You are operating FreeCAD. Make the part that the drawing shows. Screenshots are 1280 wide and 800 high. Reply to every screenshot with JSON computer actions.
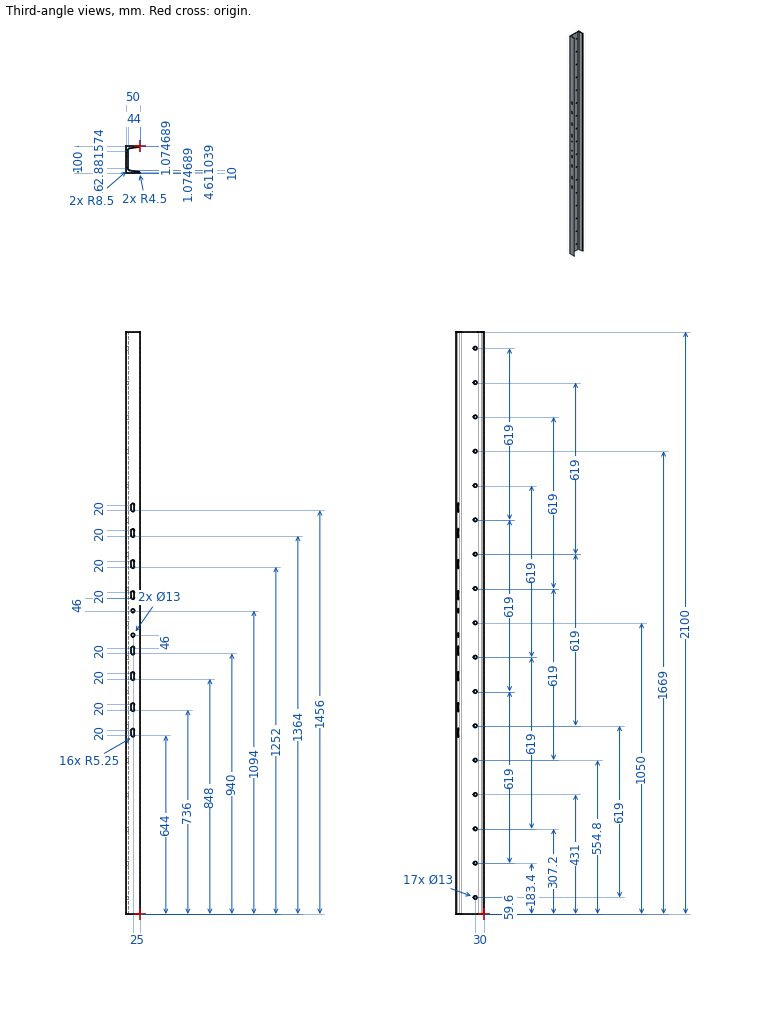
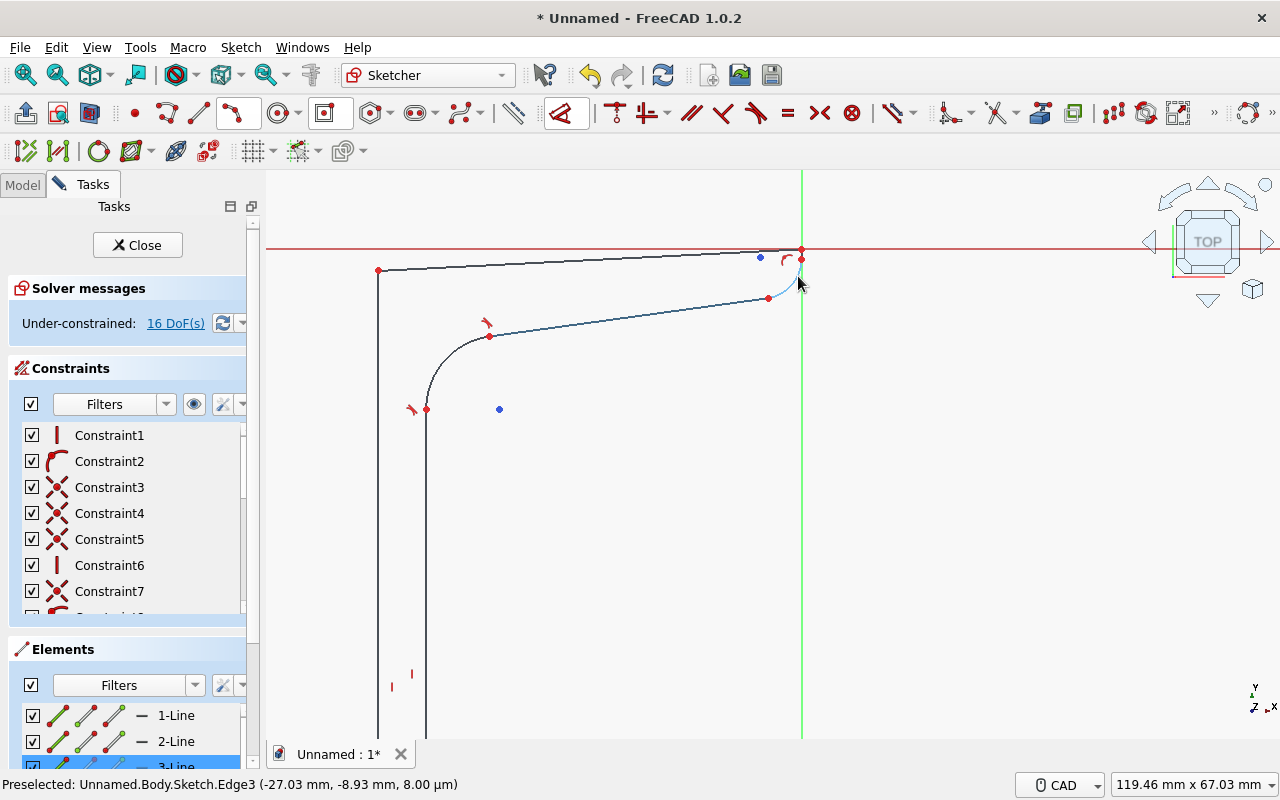
{"action": "left_click", "coordinate": [798, 275]}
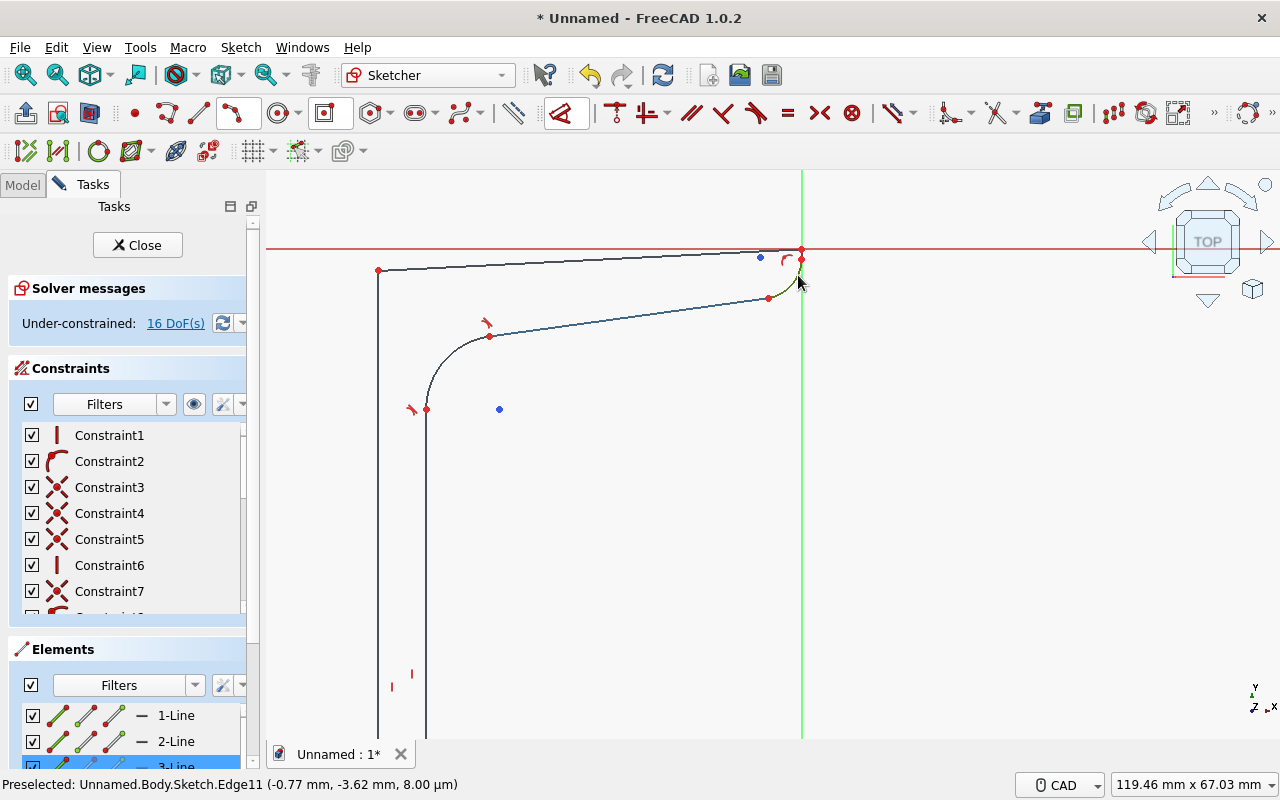
{"action": "left_click", "coordinate": [756, 114]}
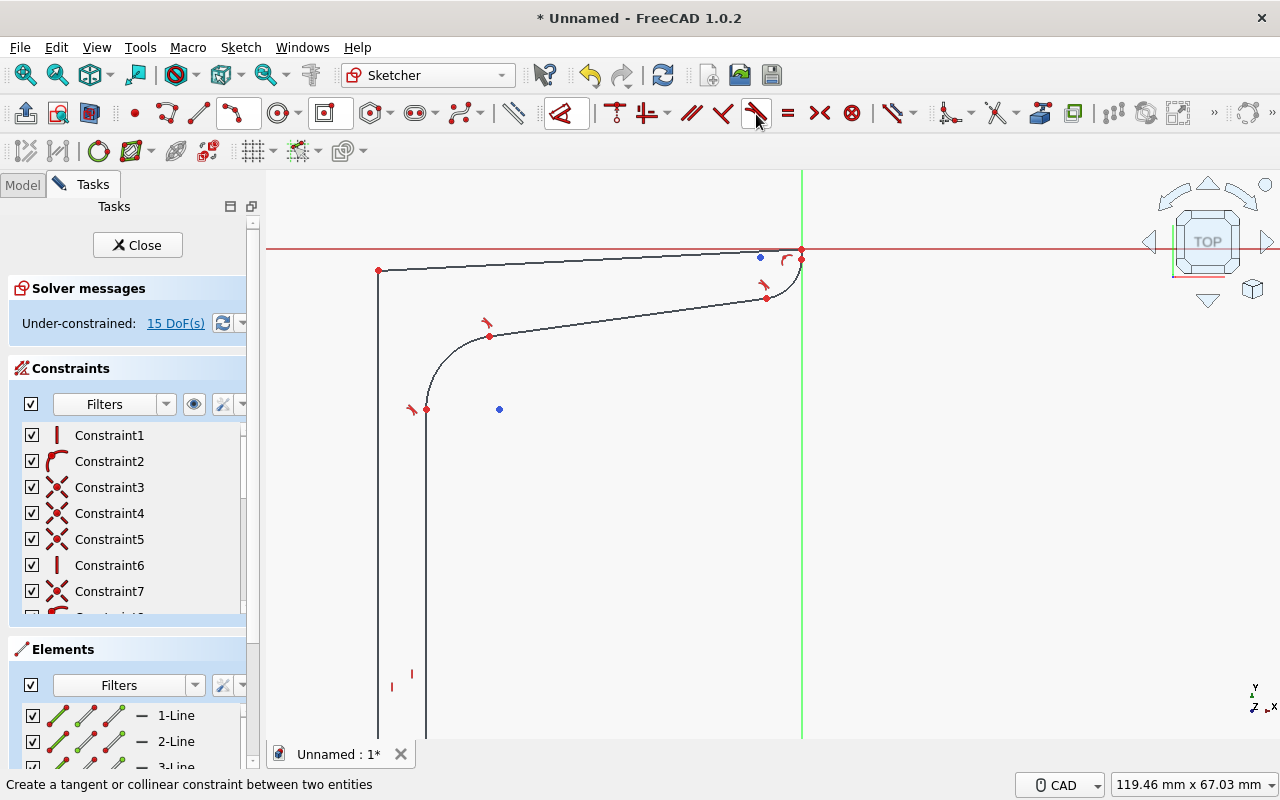
{"action": "scroll", "coordinate": [802, 254], "scroll_direction": "up", "scroll_amount": 6}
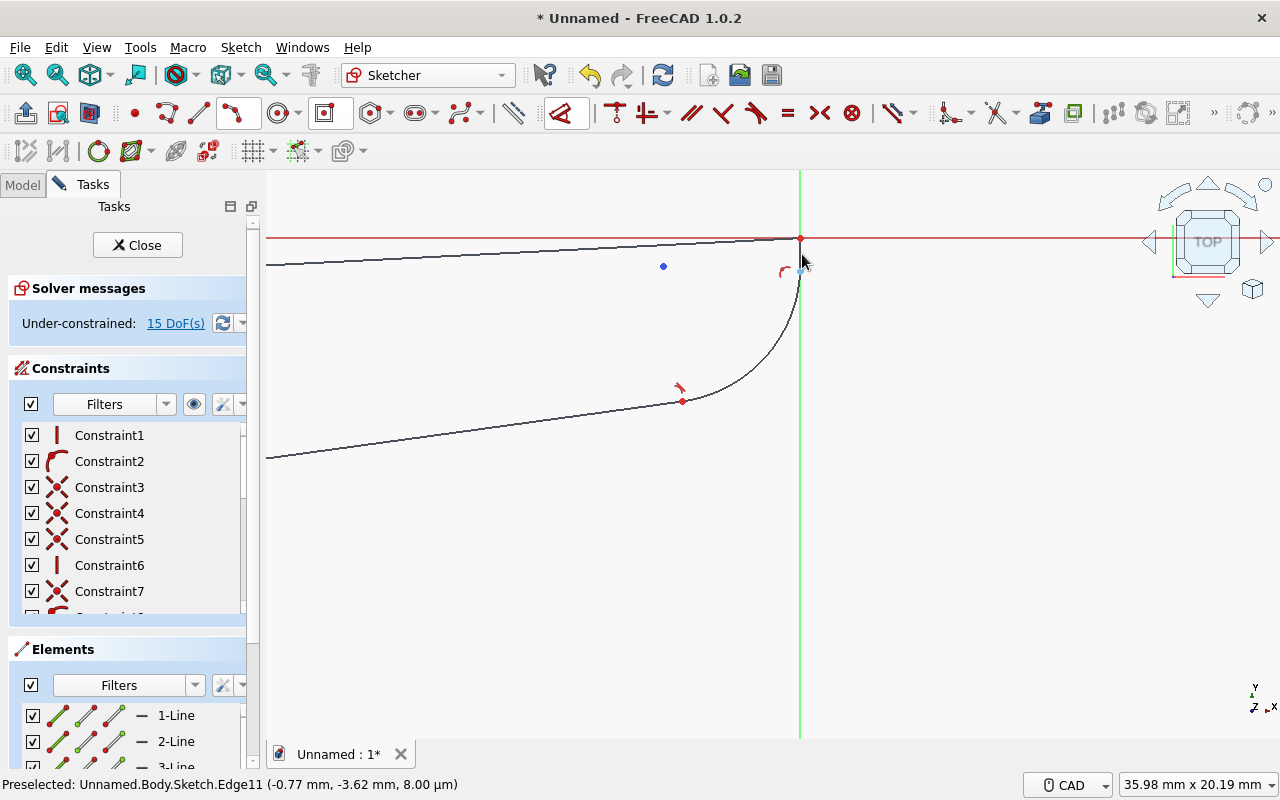
{"action": "left_click", "coordinate": [800, 255]}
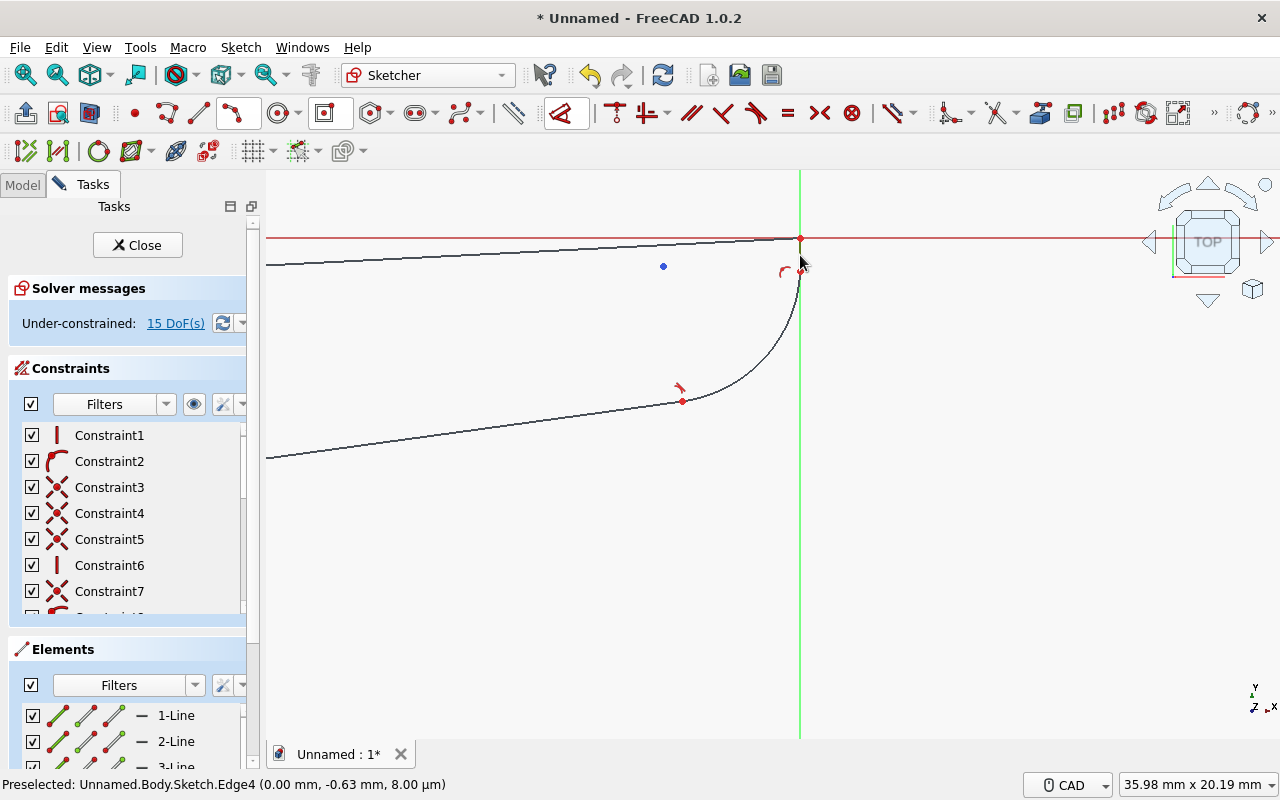
{"action": "scroll", "coordinate": [800, 268], "scroll_direction": "down", "scroll_amount": 10}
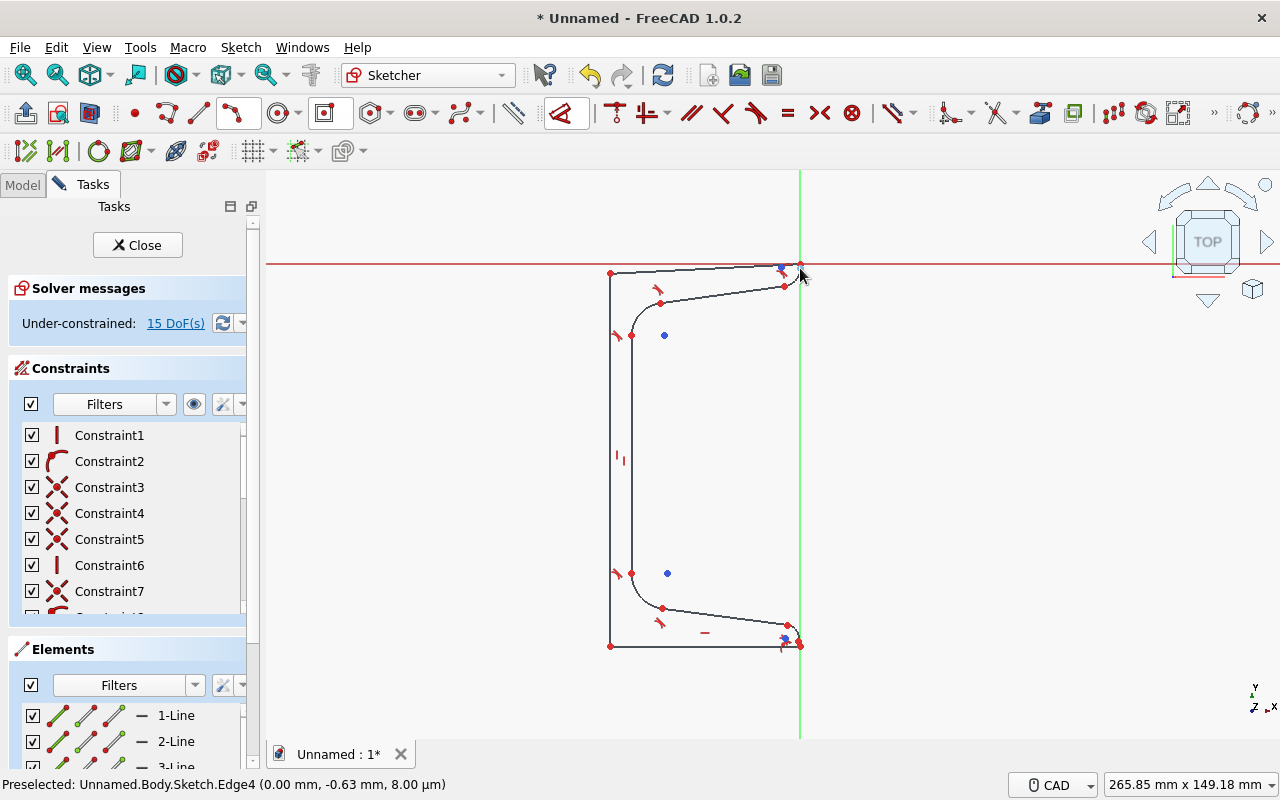
{"action": "scroll", "coordinate": [792, 284], "scroll_direction": "up", "scroll_amount": 3}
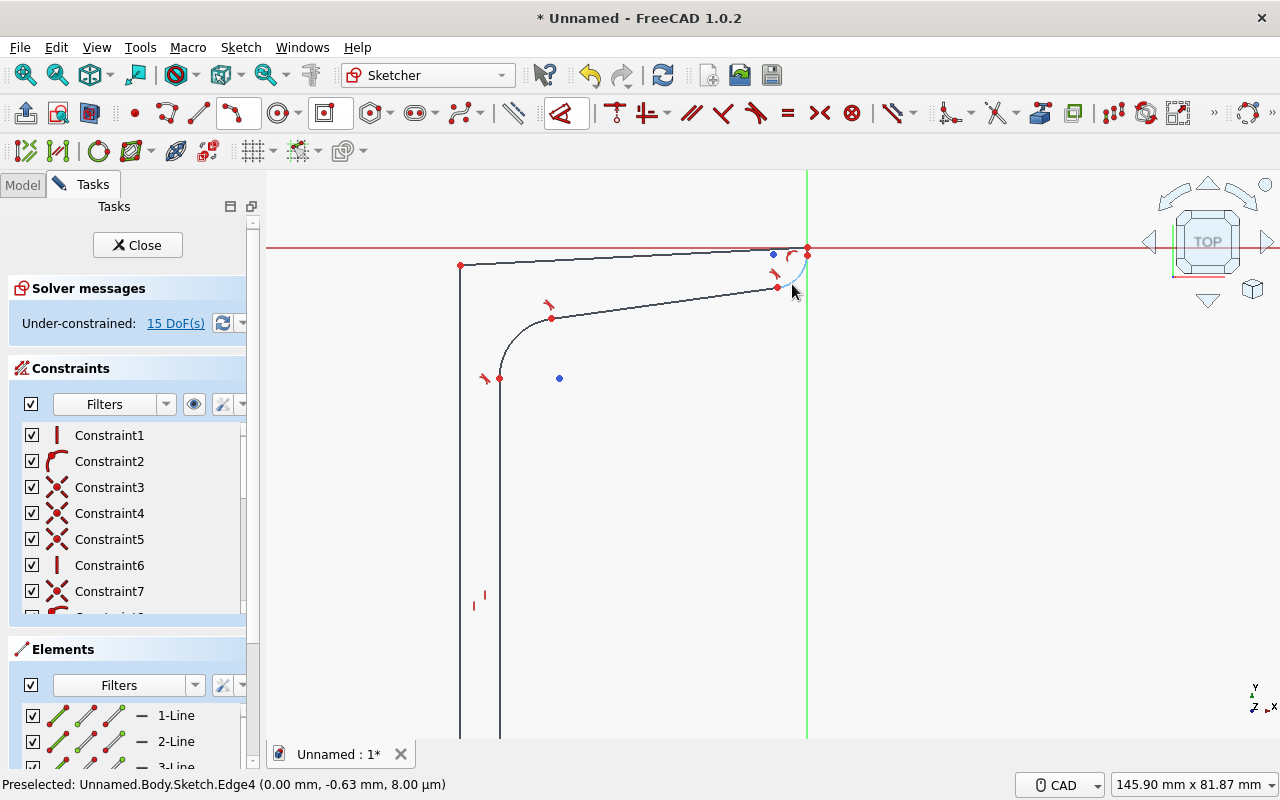
{"action": "left_click", "coordinate": [791, 283]}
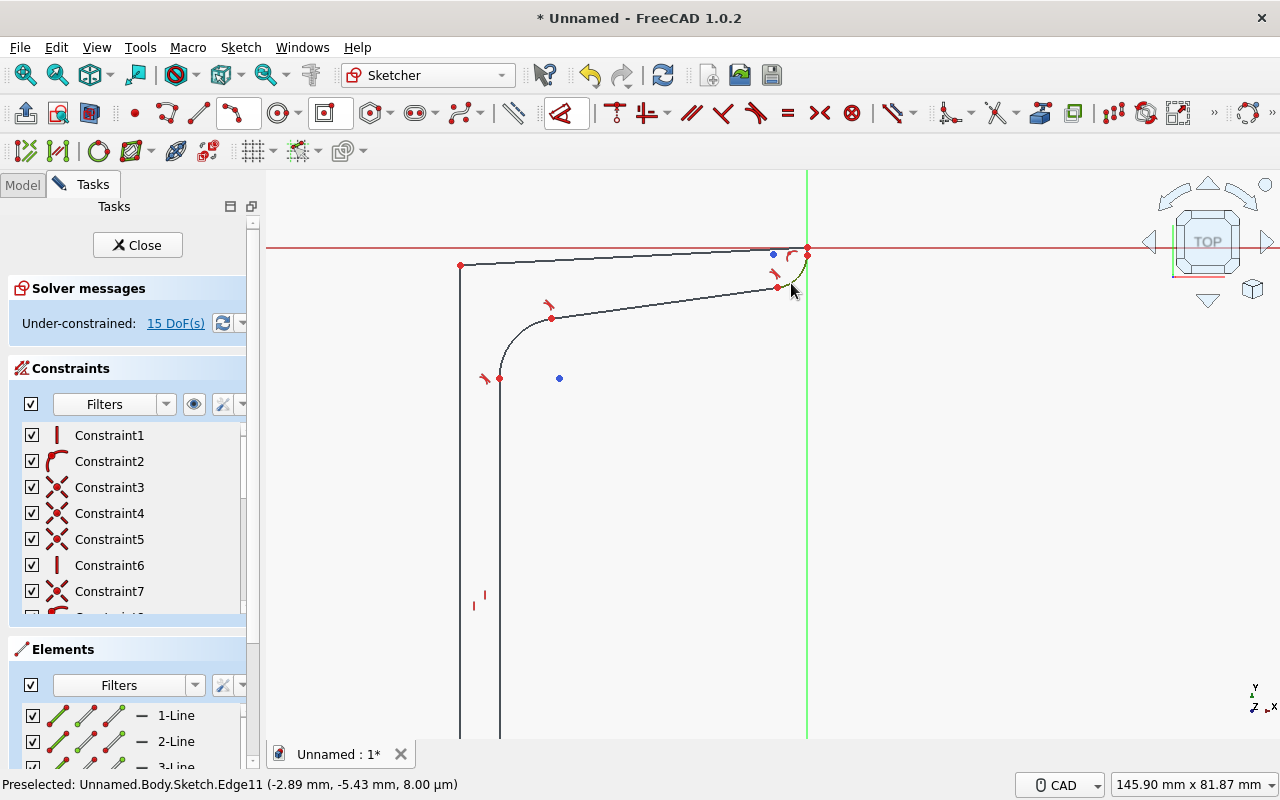
{"action": "key", "text": "t"}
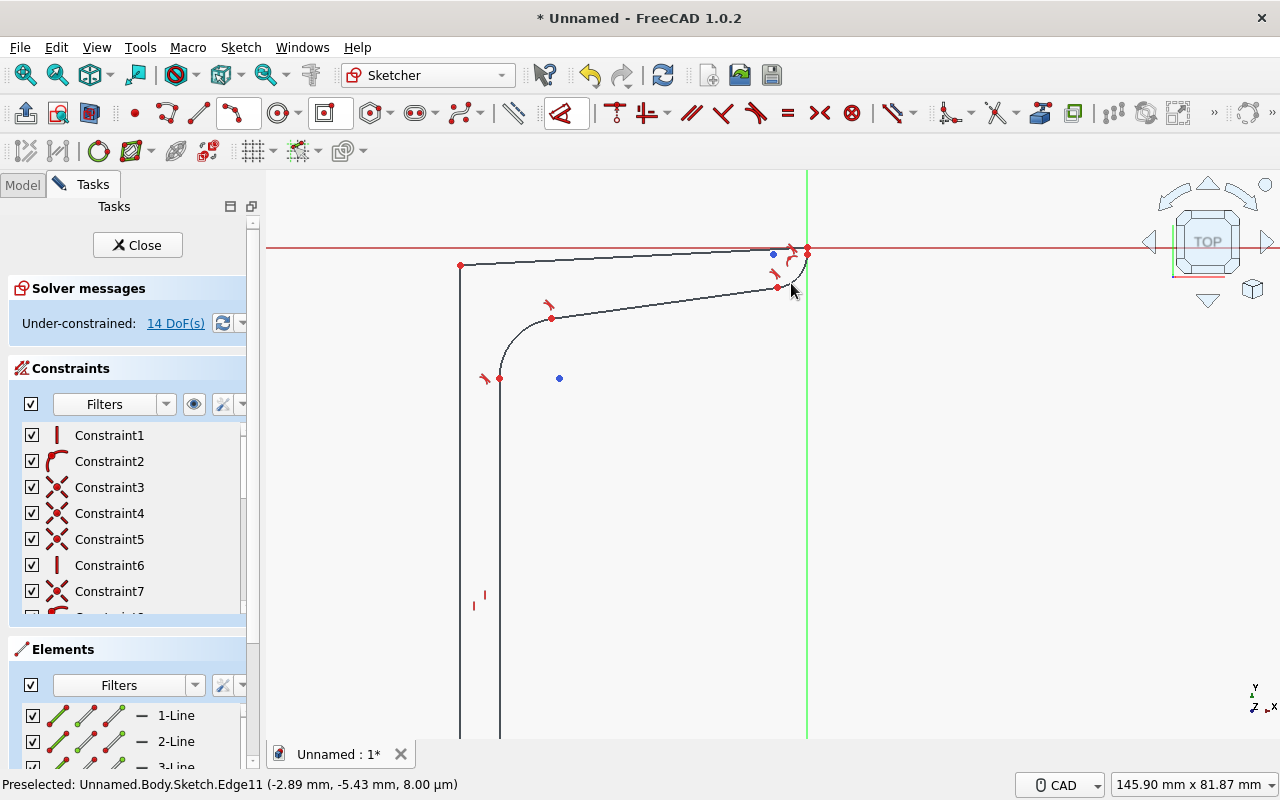
{"action": "scroll", "coordinate": [791, 283], "scroll_direction": "down", "scroll_amount": 3}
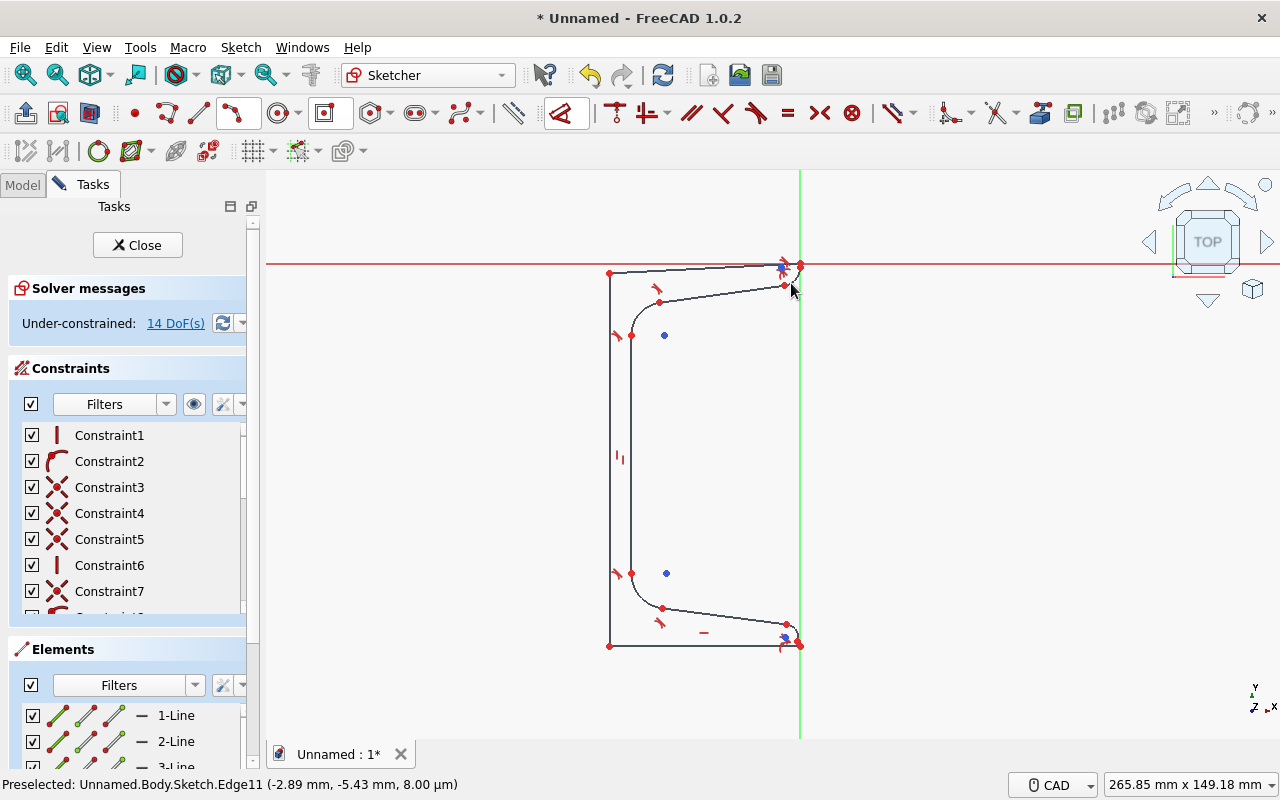
{"action": "scroll", "coordinate": [799, 644], "scroll_direction": "up", "scroll_amount": 9}